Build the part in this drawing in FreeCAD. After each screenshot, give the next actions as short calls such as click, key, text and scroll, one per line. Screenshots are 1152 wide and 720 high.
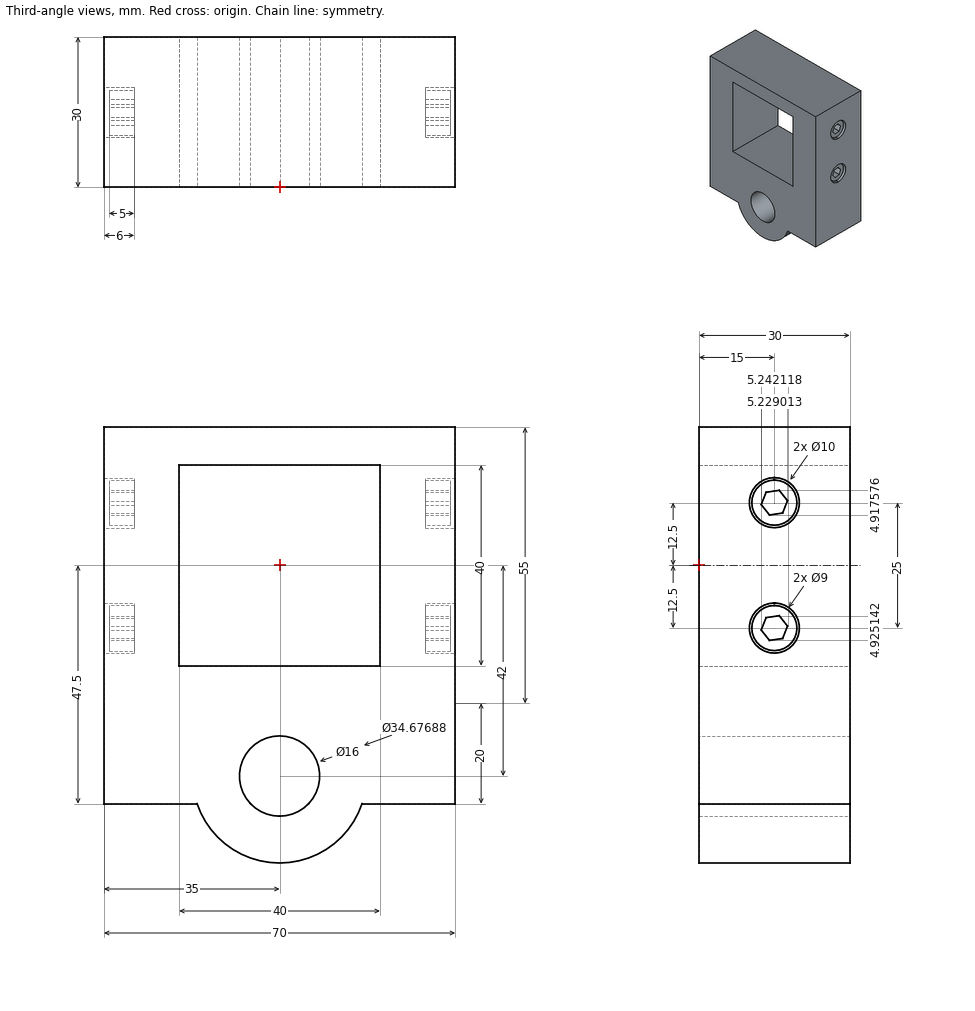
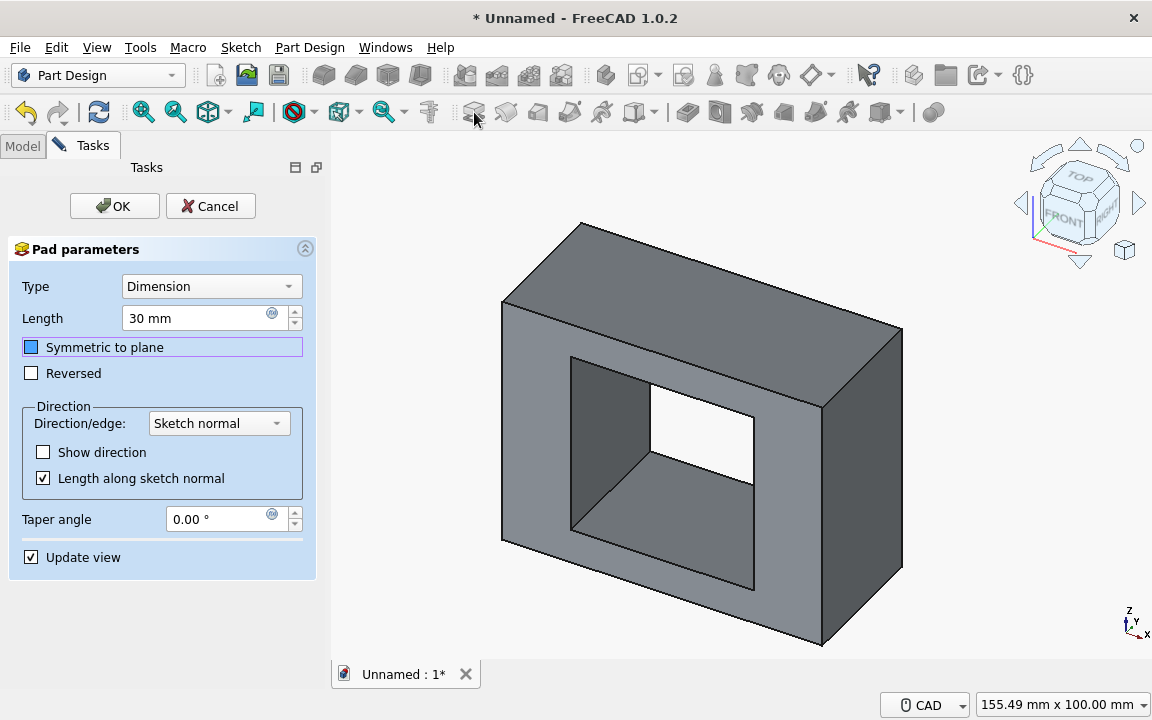
click(30, 373)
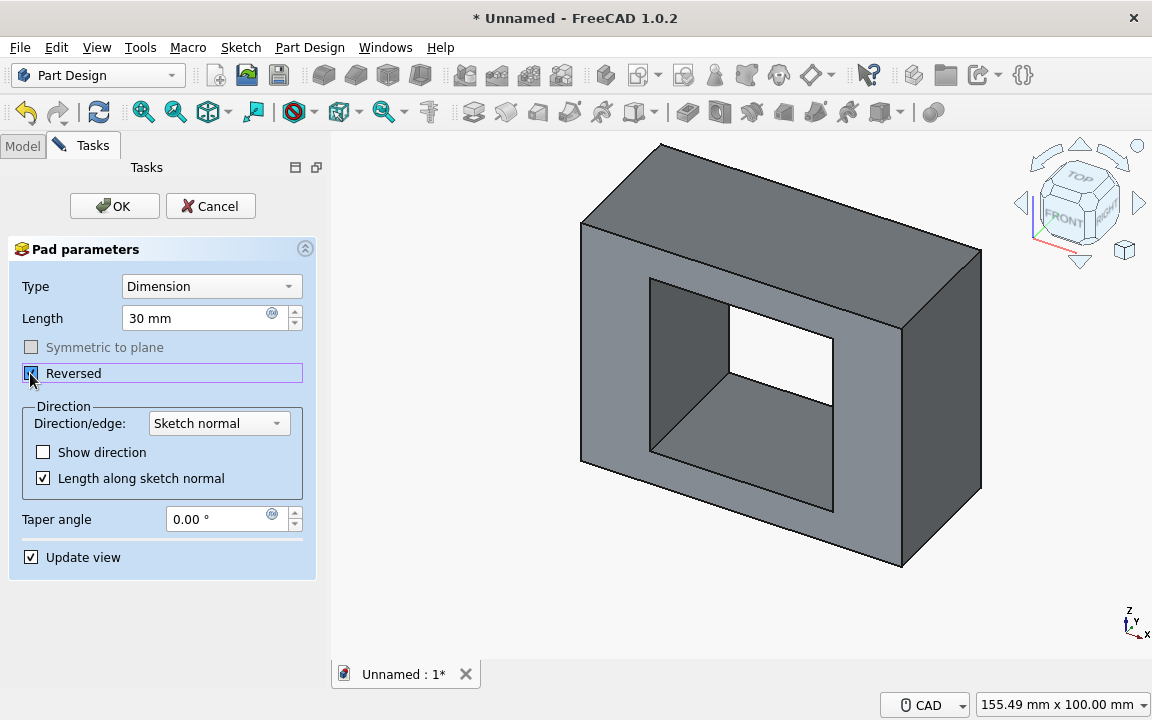
click(115, 206)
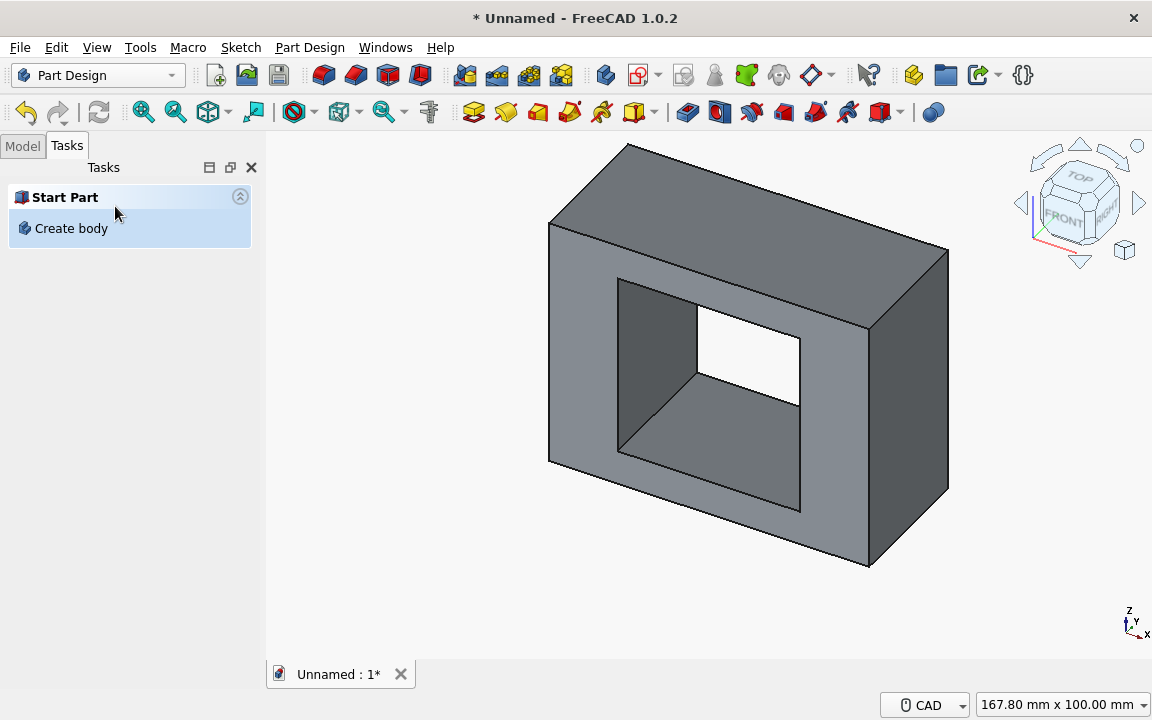
key(4)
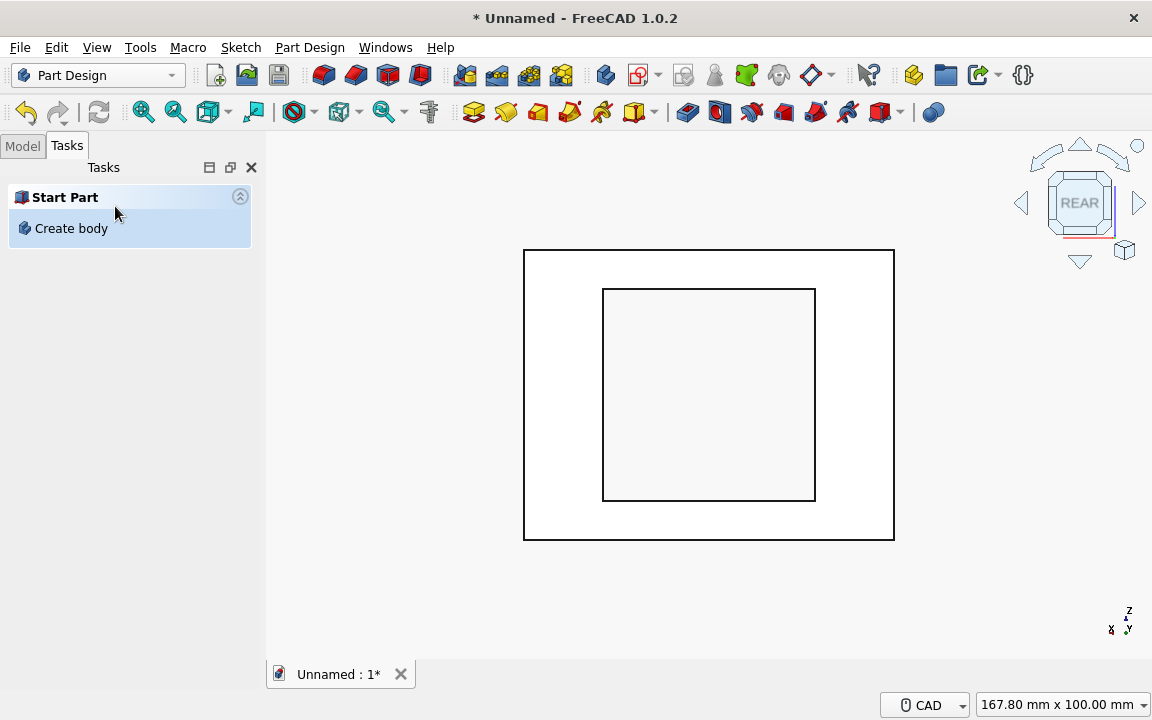
click(551, 311)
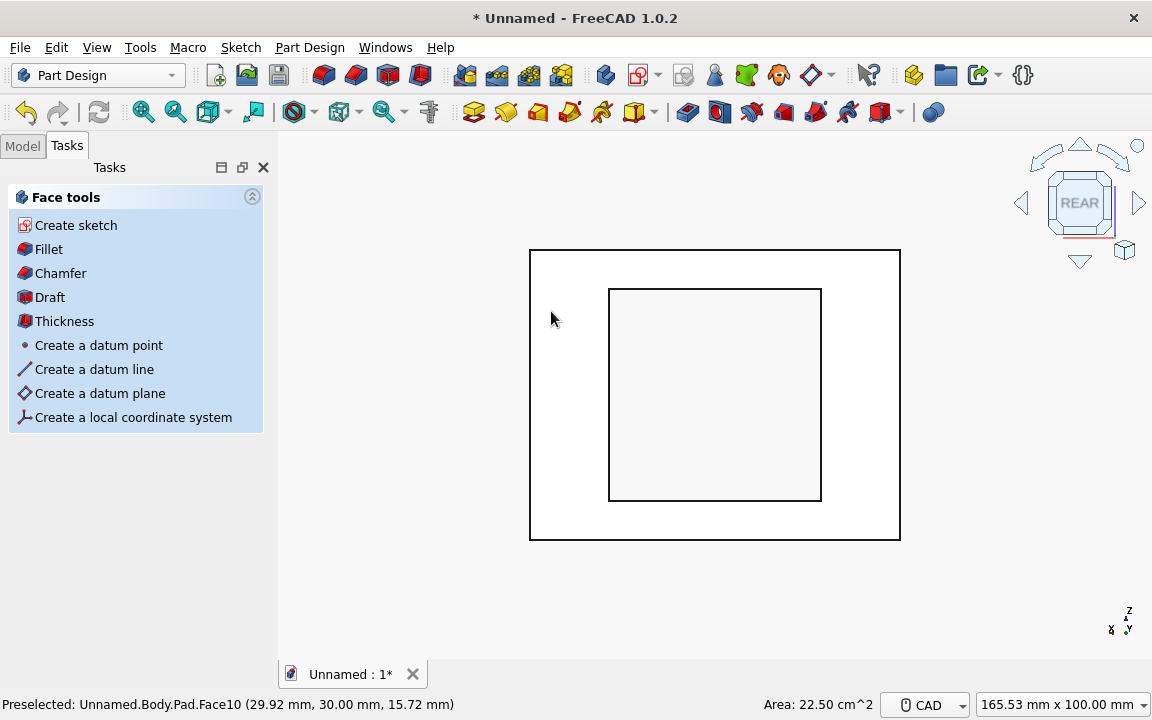
click(638, 76)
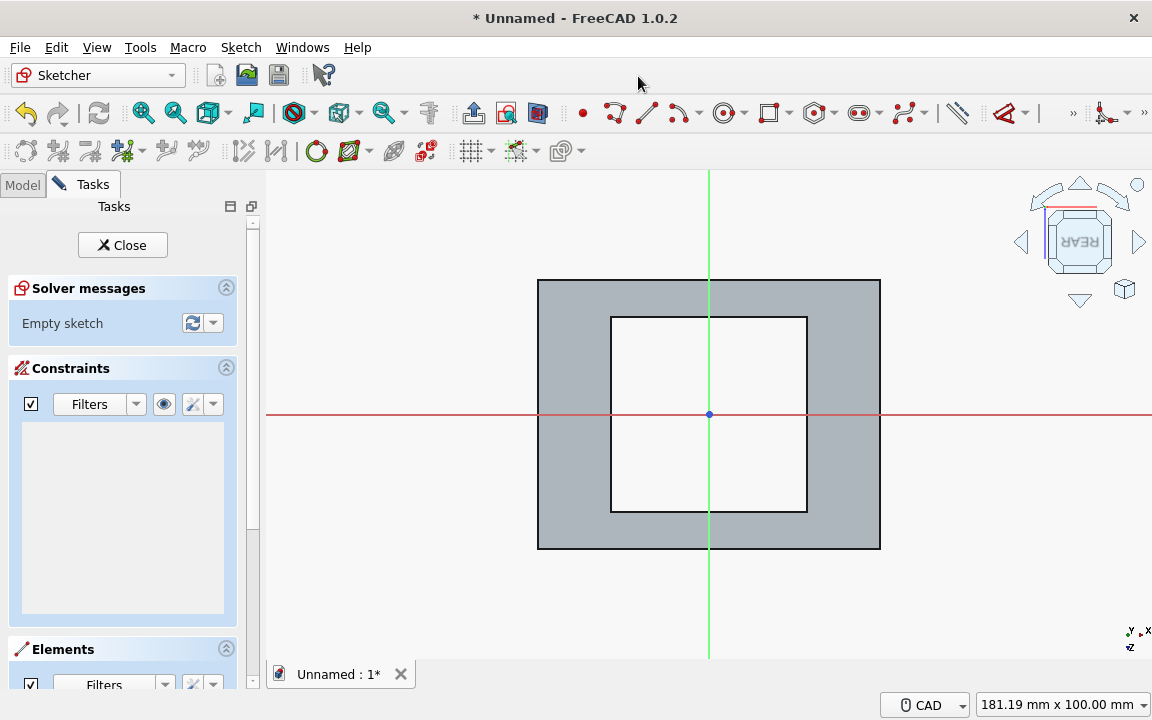
scroll(331, 631, down, 1)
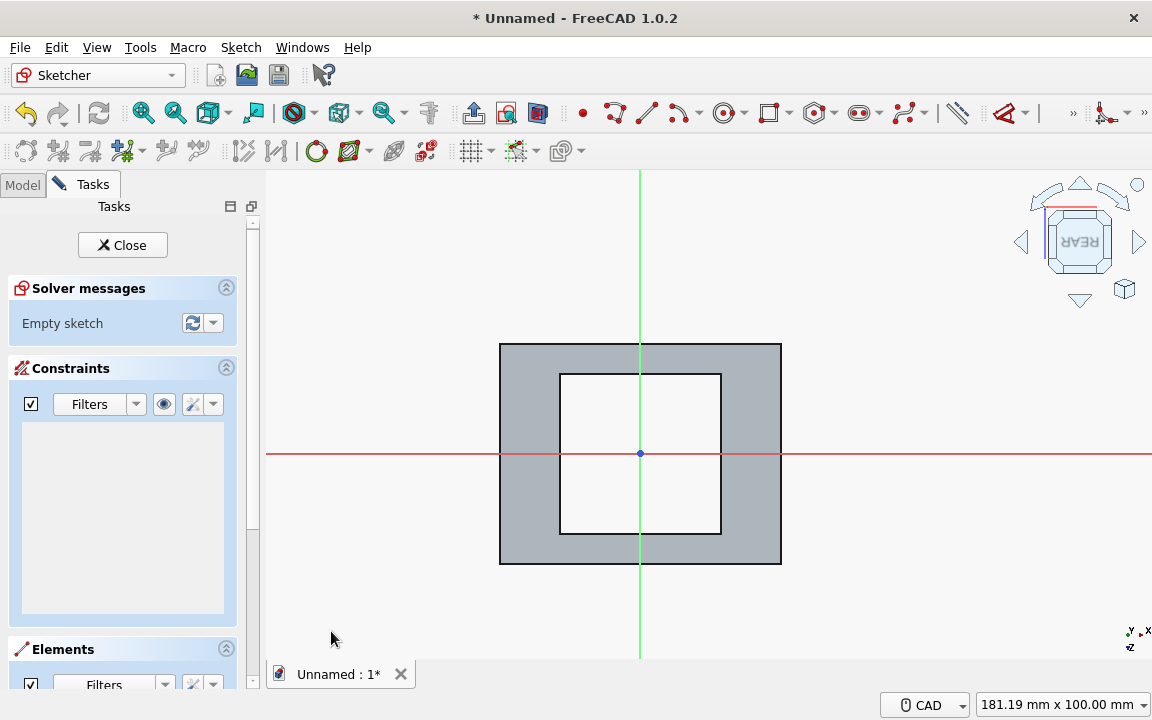
scroll(640, 246, up, 2)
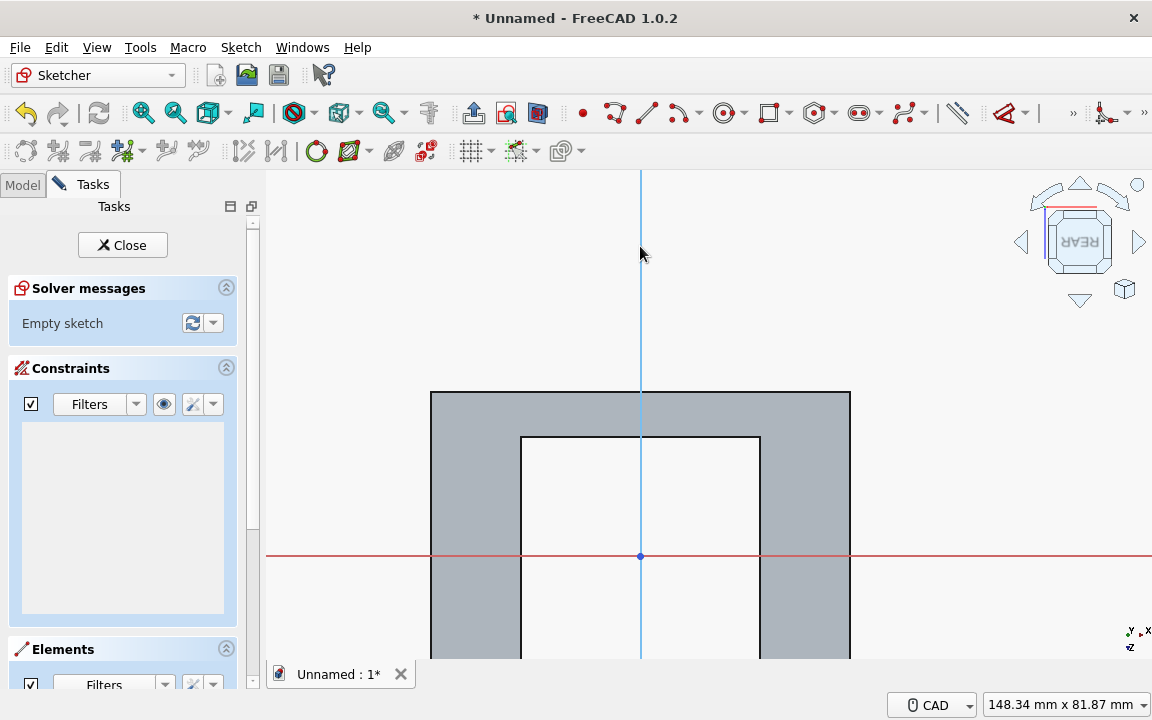
click(770, 114)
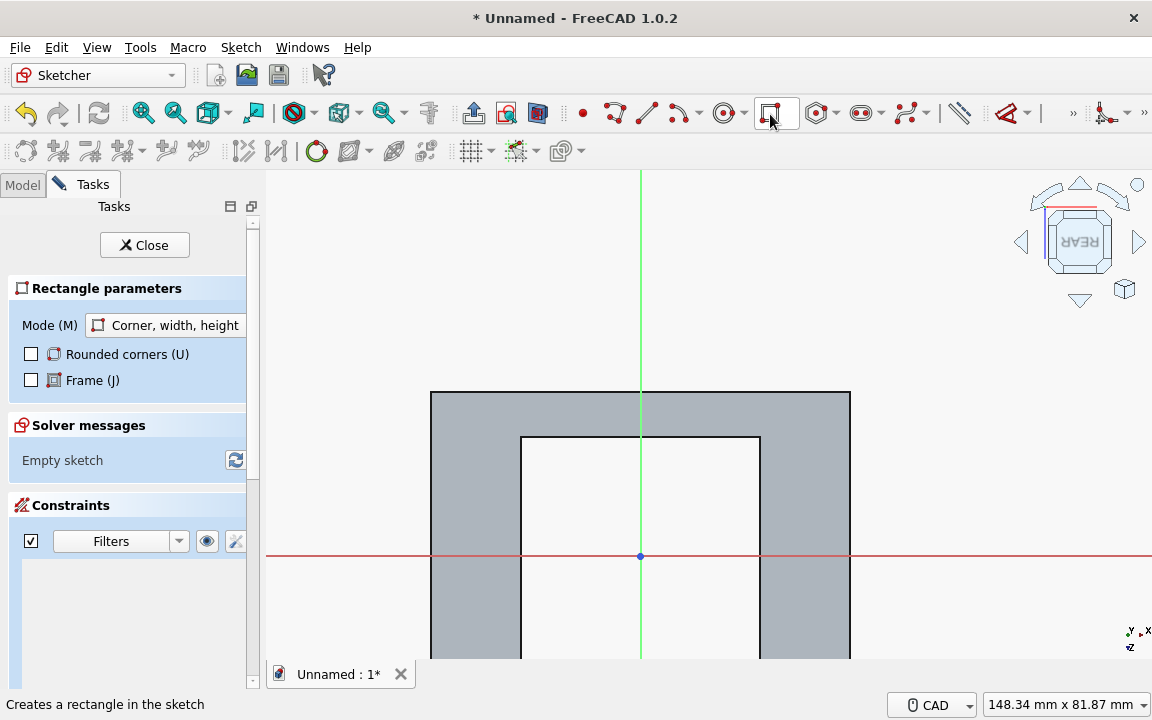
click(431, 272)
move(850, 392)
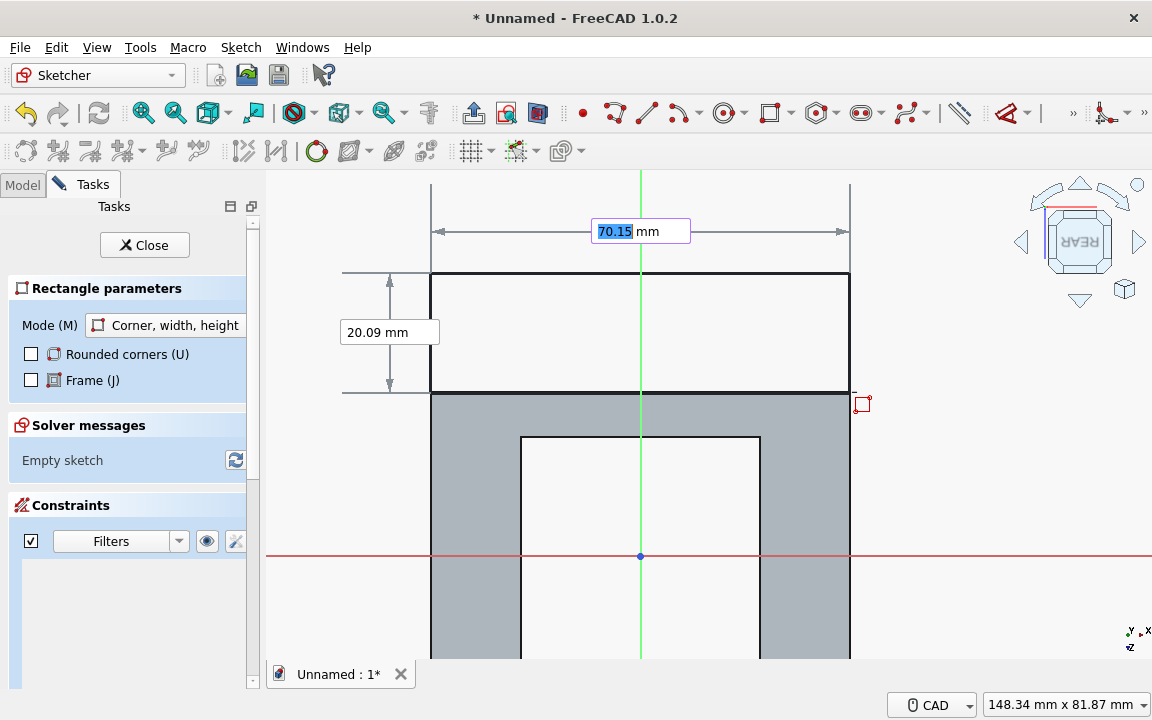
text(70)
key(Tab)
text(20)
key(Return)
key(Escape)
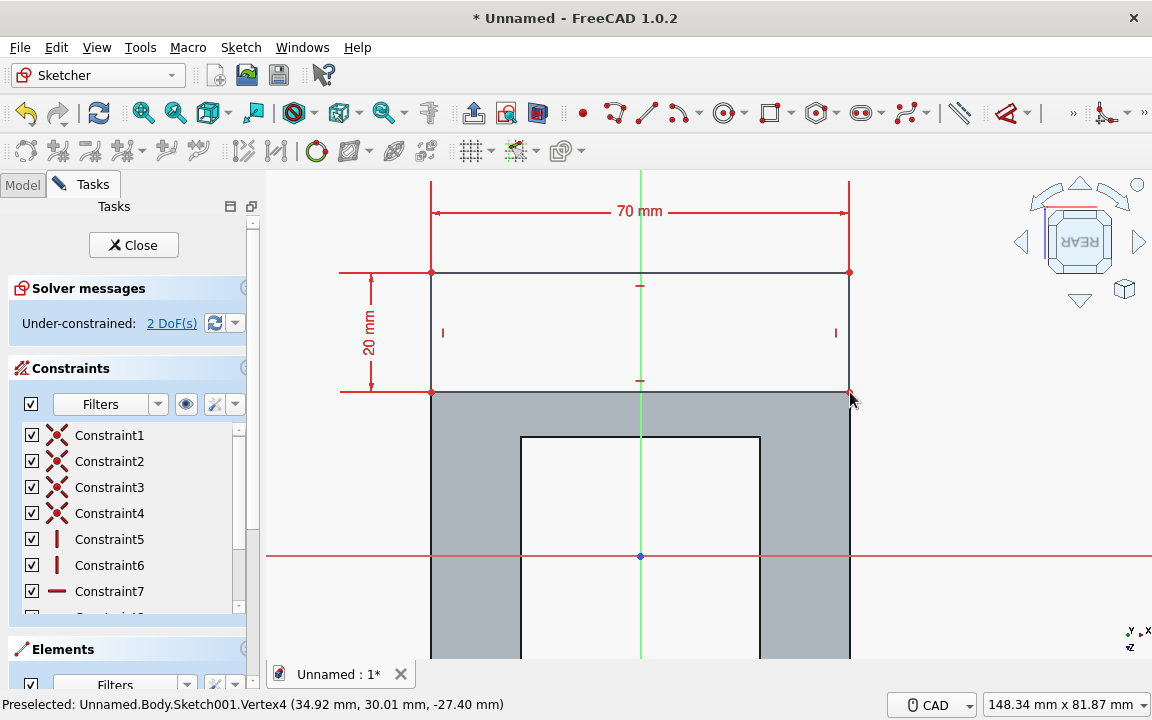
click(1006, 114)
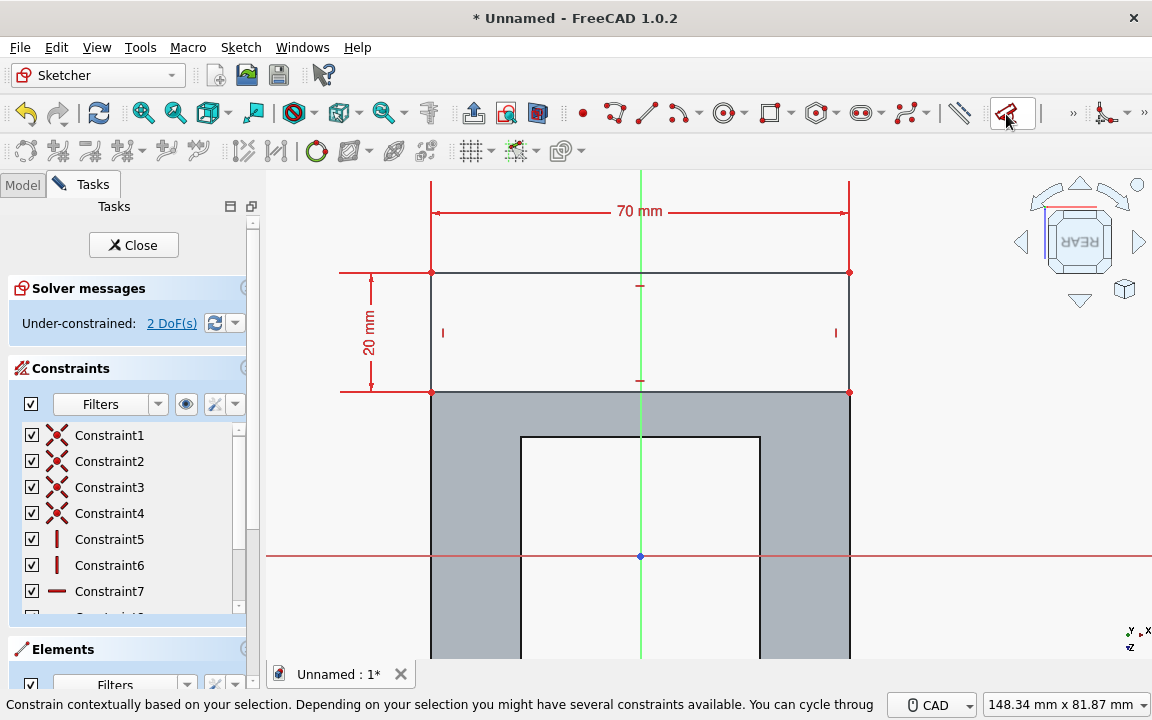
click(431, 273)
click(536, 590)